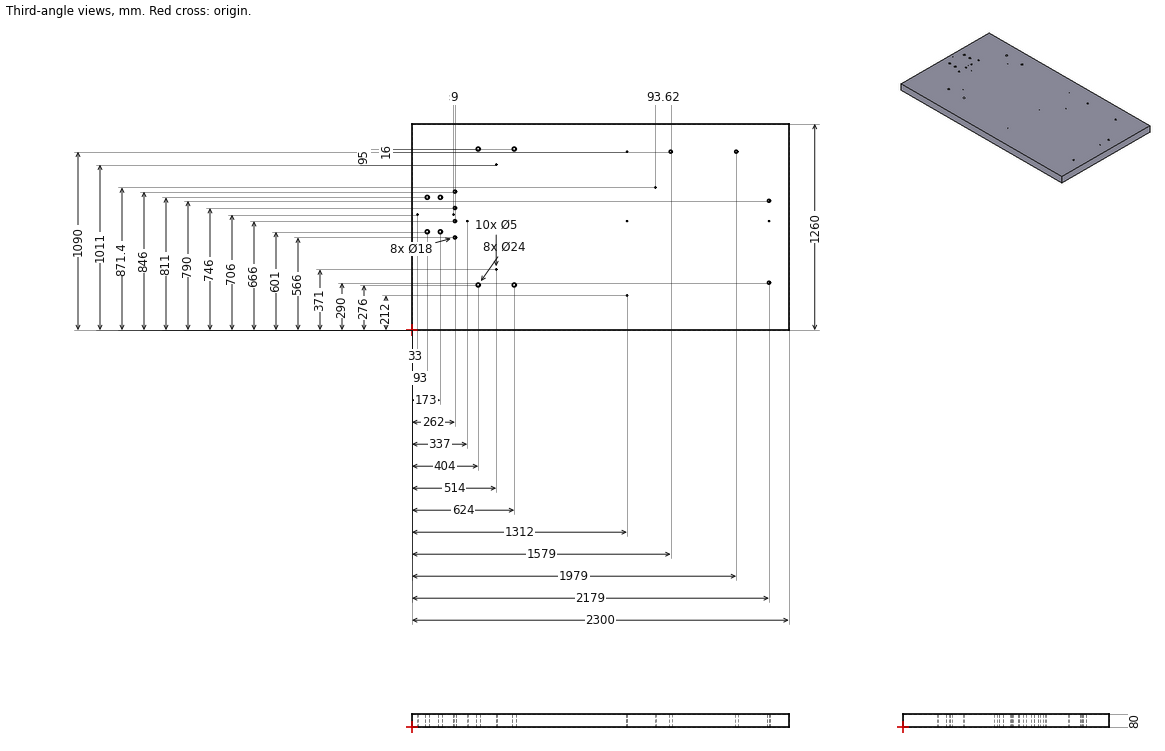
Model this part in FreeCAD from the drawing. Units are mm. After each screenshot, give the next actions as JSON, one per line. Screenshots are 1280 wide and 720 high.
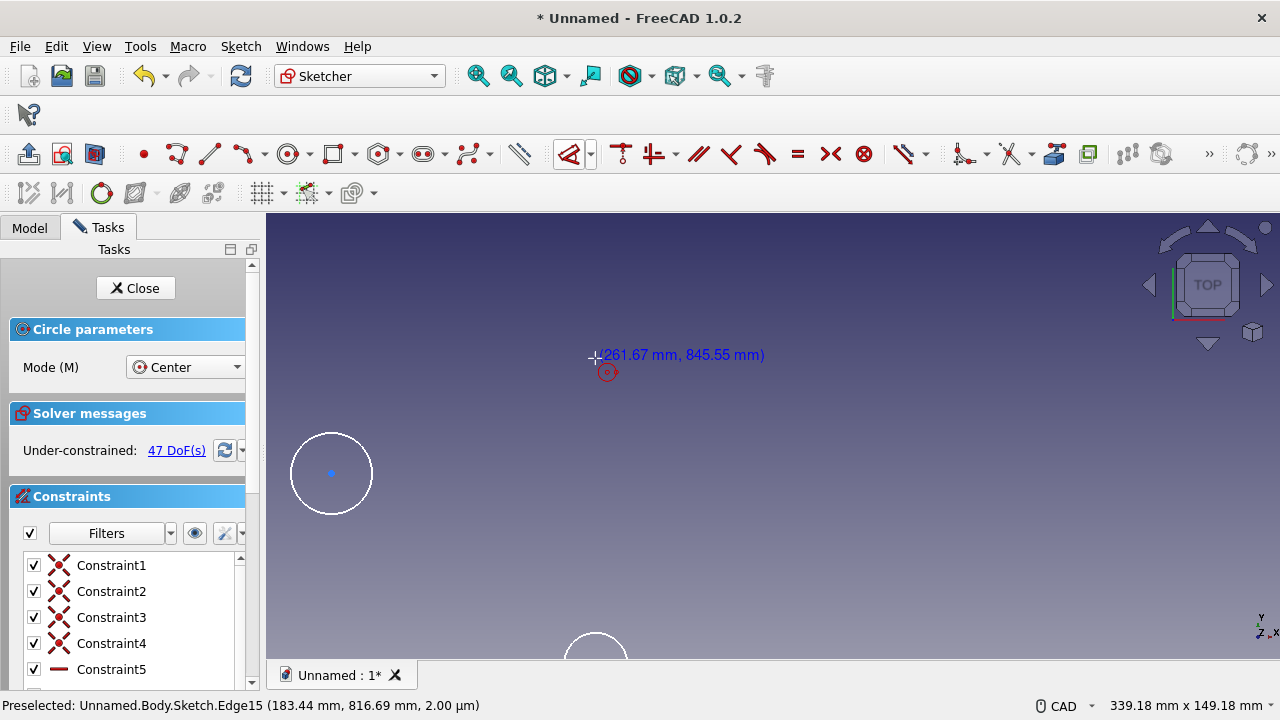
{"action": "scroll", "coordinate": [500, 390], "scroll_direction": "down", "scroll_amount": 13}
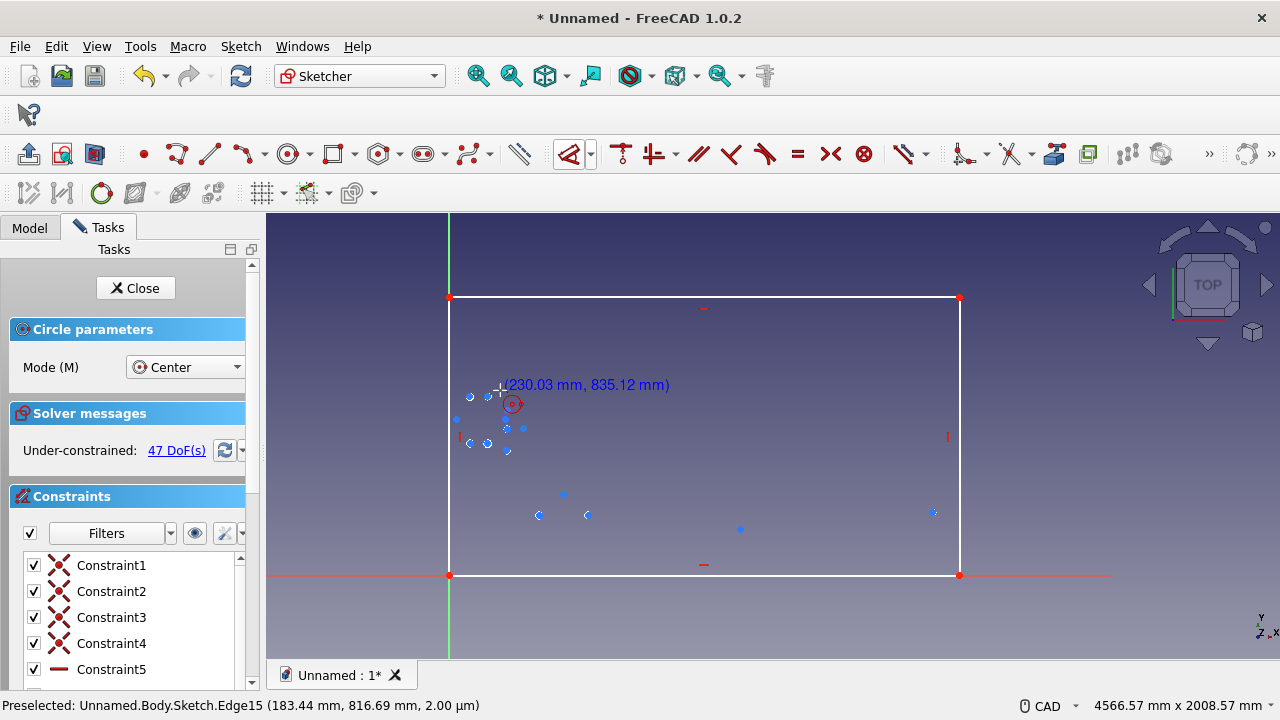
{"action": "left_click", "coordinate": [507, 388]}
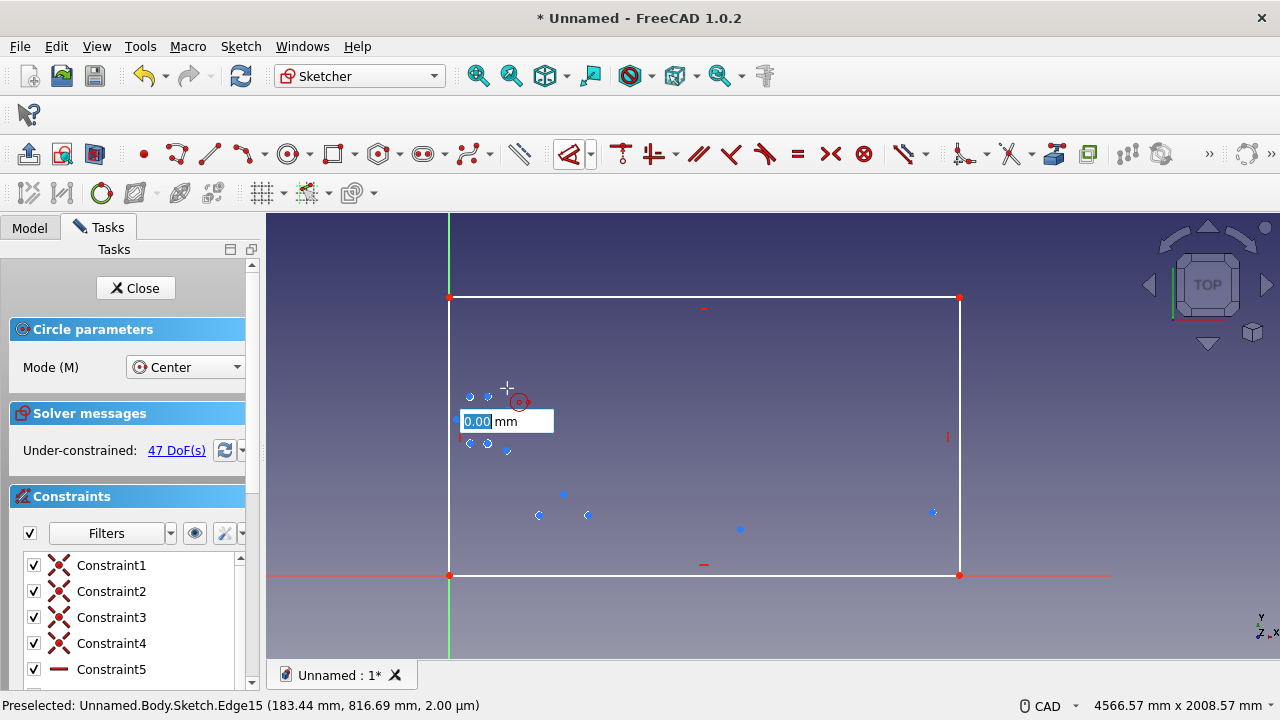
{"action": "scroll", "coordinate": [509, 387], "scroll_direction": "up", "scroll_amount": 11}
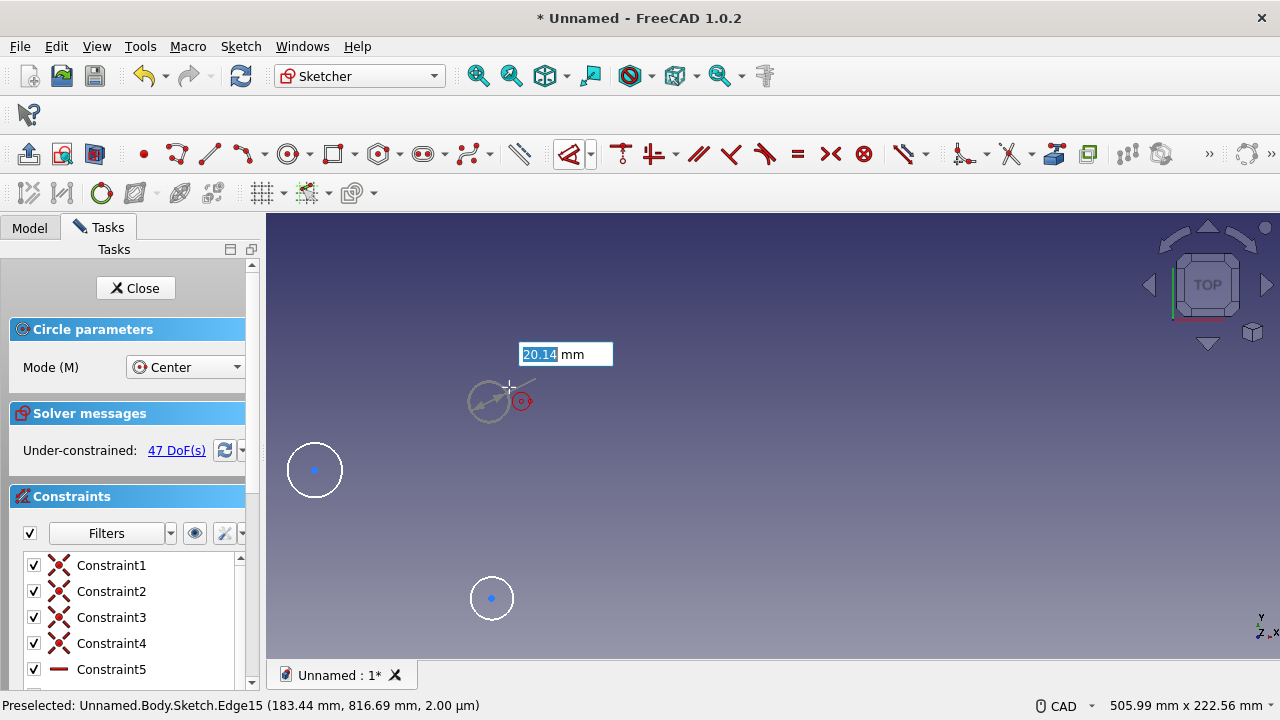
{"action": "left_click", "coordinate": [505, 380]}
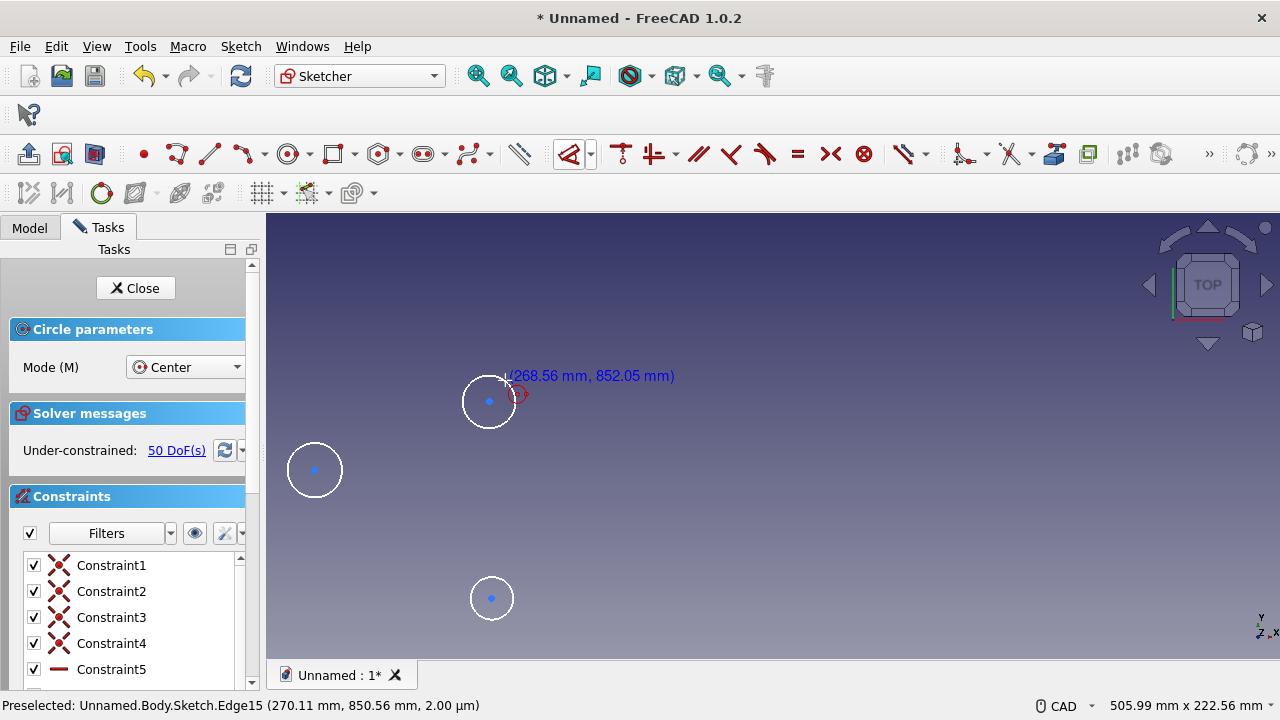
{"action": "scroll", "coordinate": [509, 387], "scroll_direction": "down", "scroll_amount": 11}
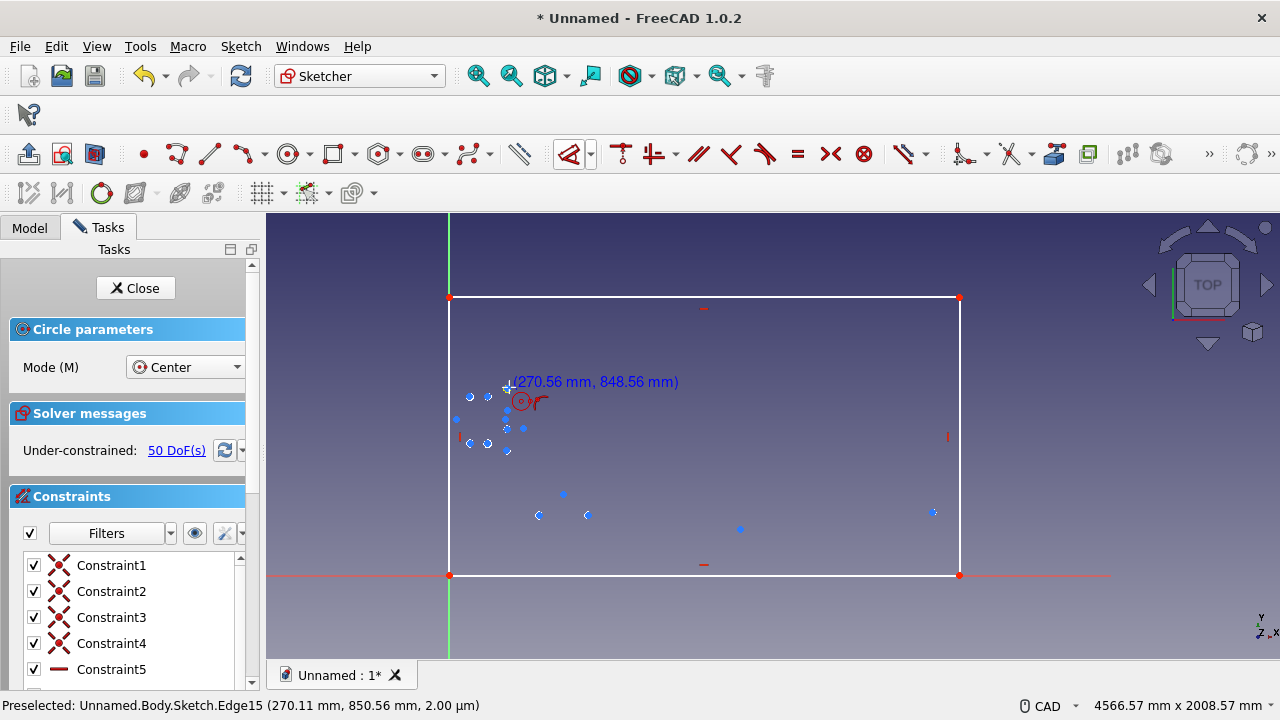
{"action": "scroll", "coordinate": [563, 351], "scroll_direction": "up", "scroll_amount": 19}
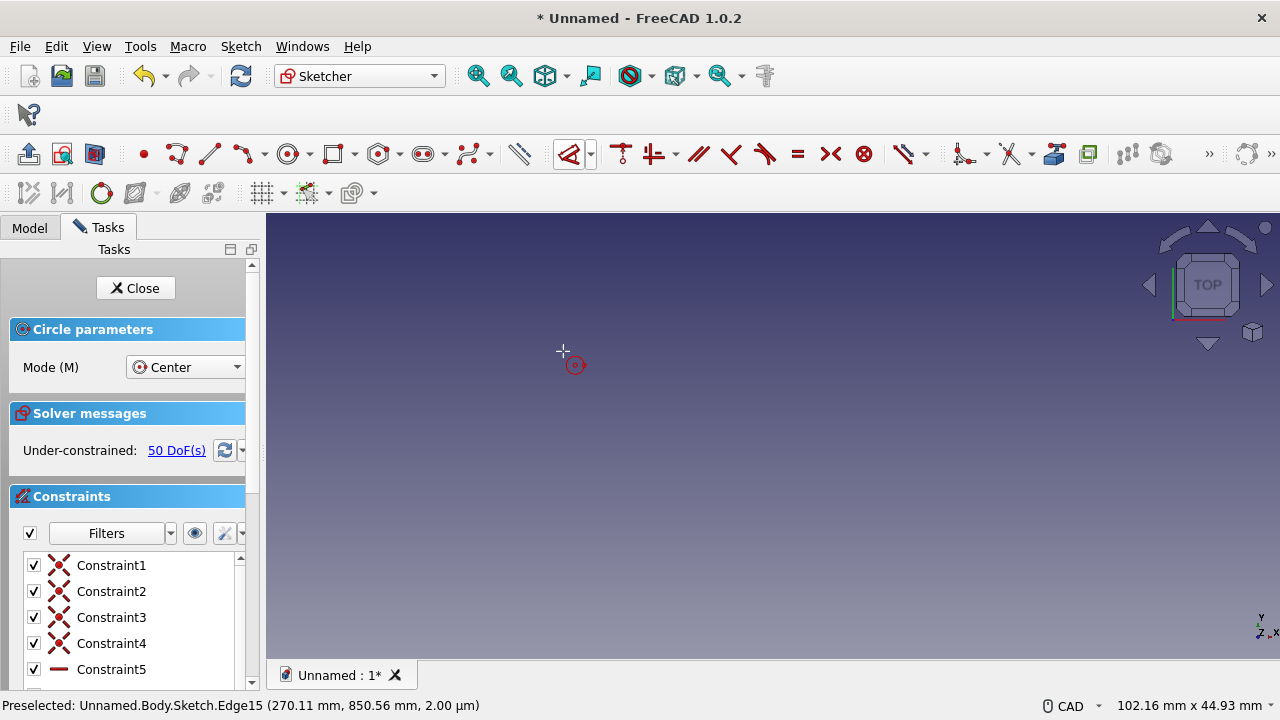
{"action": "scroll", "coordinate": [704, 436], "scroll_direction": "down", "scroll_amount": 15}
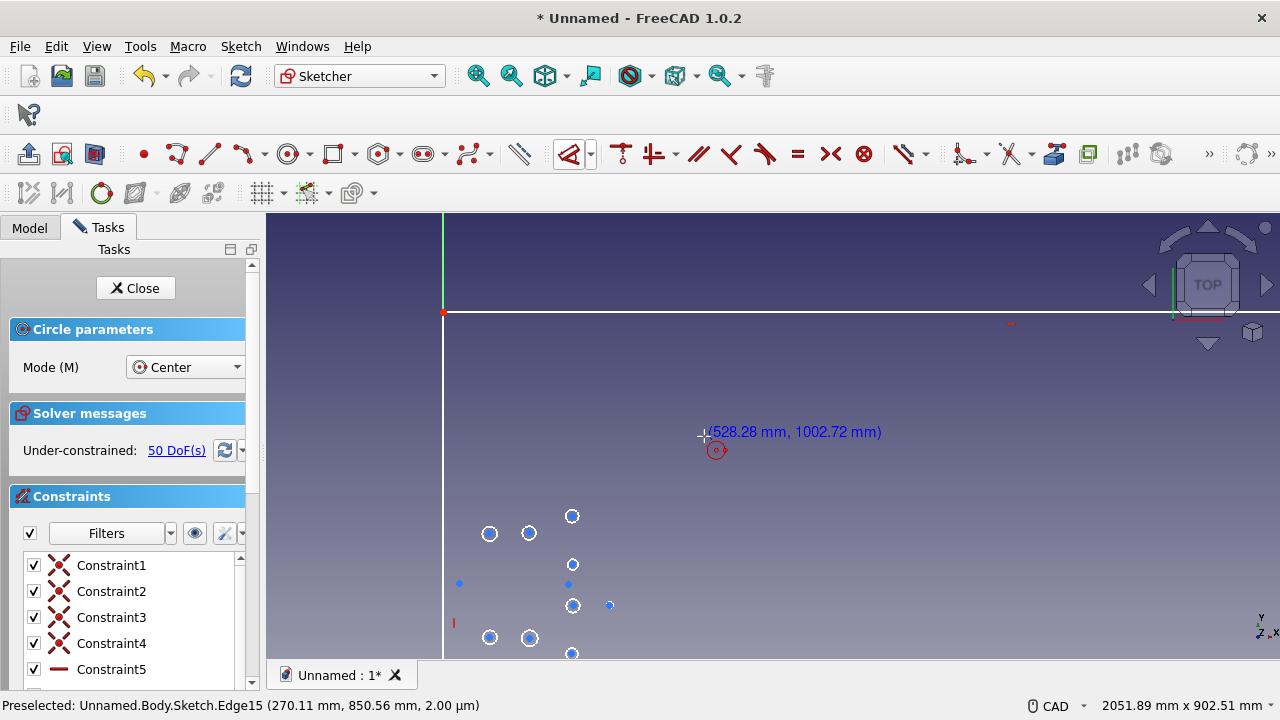
{"action": "scroll", "coordinate": [454, 285], "scroll_direction": "down", "scroll_amount": 4}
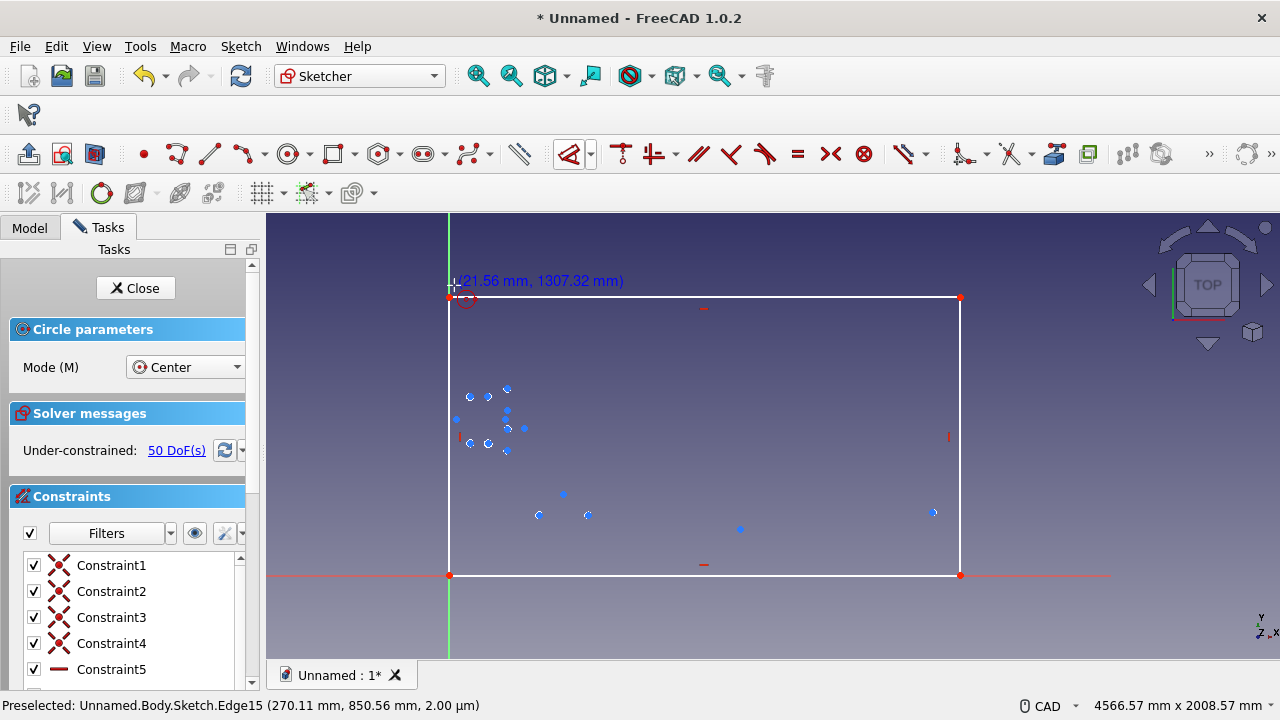
{"action": "left_click", "coordinate": [563, 351]}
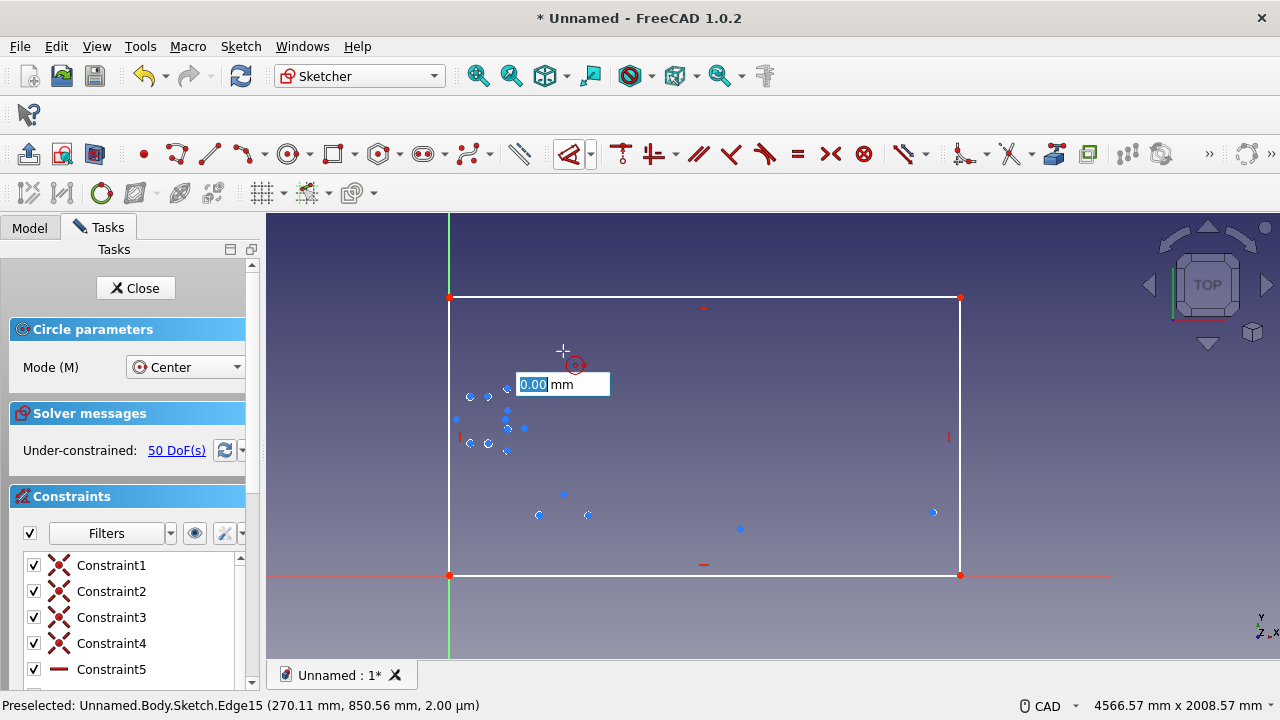
{"action": "scroll", "coordinate": [564, 351], "scroll_direction": "up", "scroll_amount": 17}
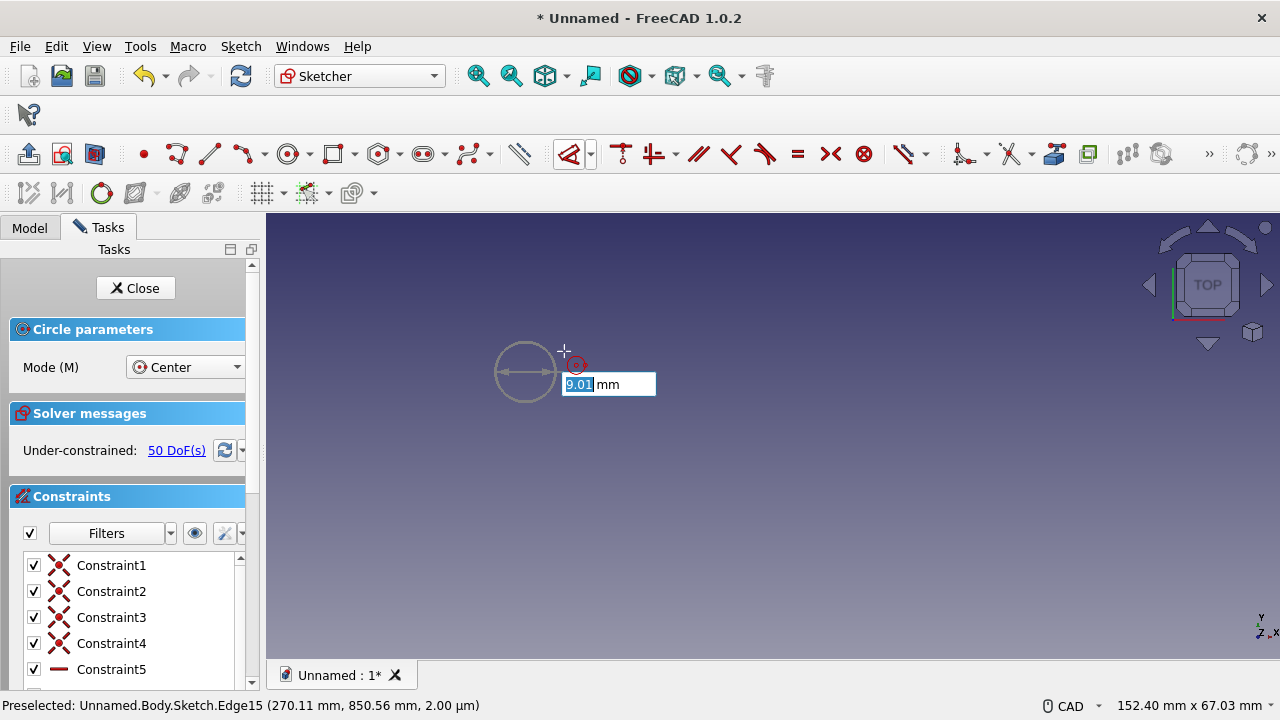
{"action": "left_click", "coordinate": [551, 340]}